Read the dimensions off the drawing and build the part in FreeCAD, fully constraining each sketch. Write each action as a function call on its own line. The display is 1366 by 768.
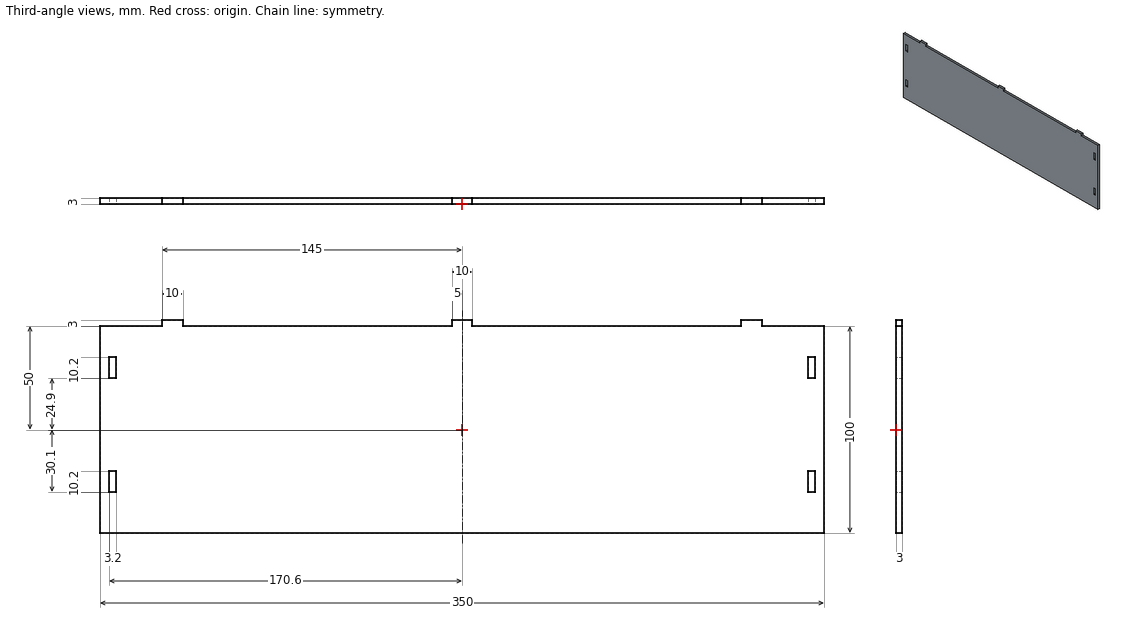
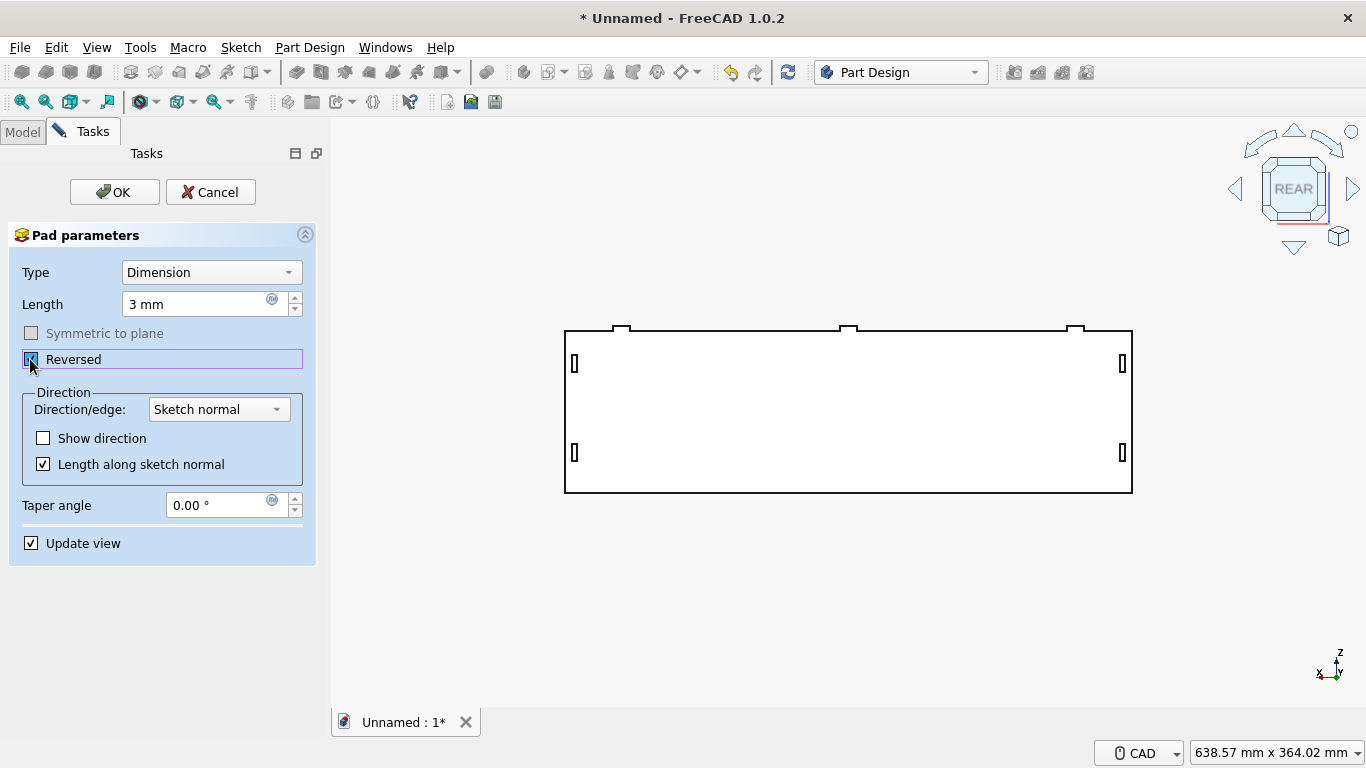
click(115, 192)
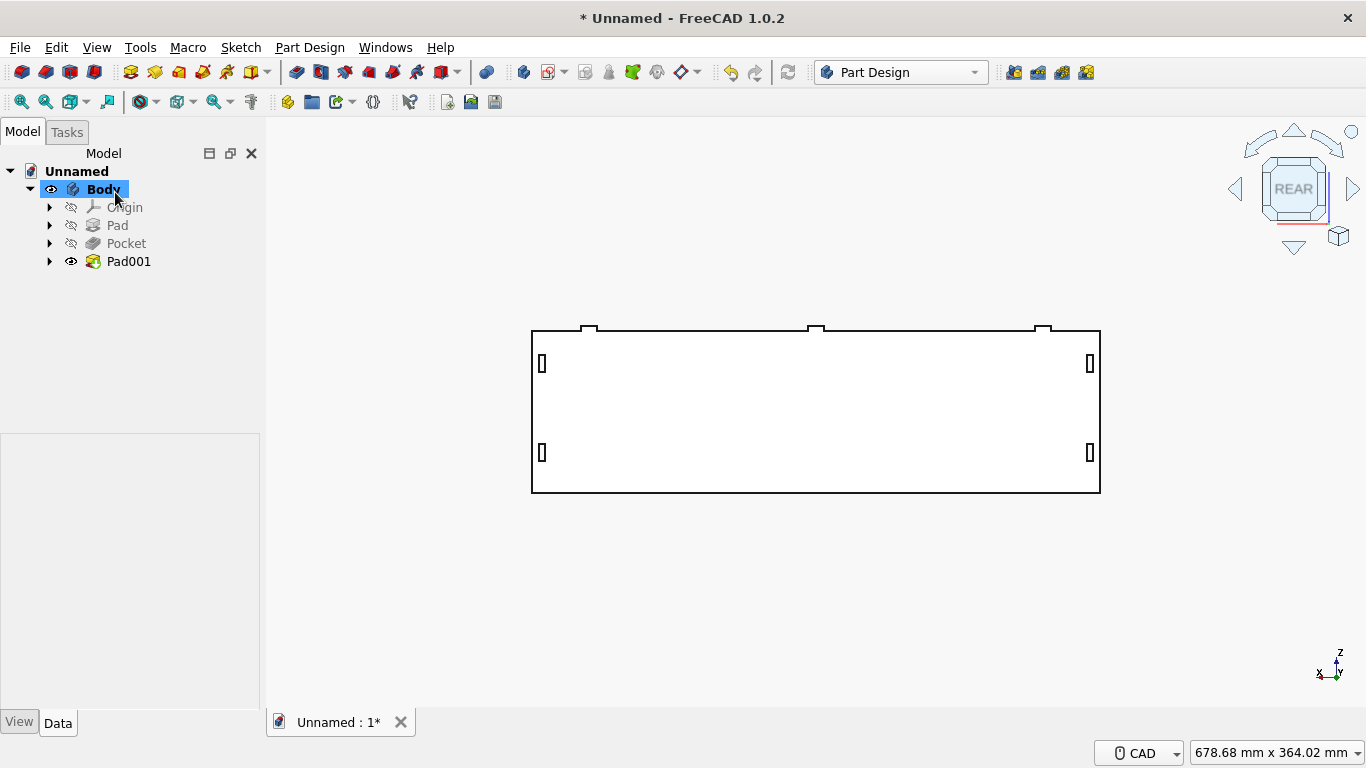
key(0)